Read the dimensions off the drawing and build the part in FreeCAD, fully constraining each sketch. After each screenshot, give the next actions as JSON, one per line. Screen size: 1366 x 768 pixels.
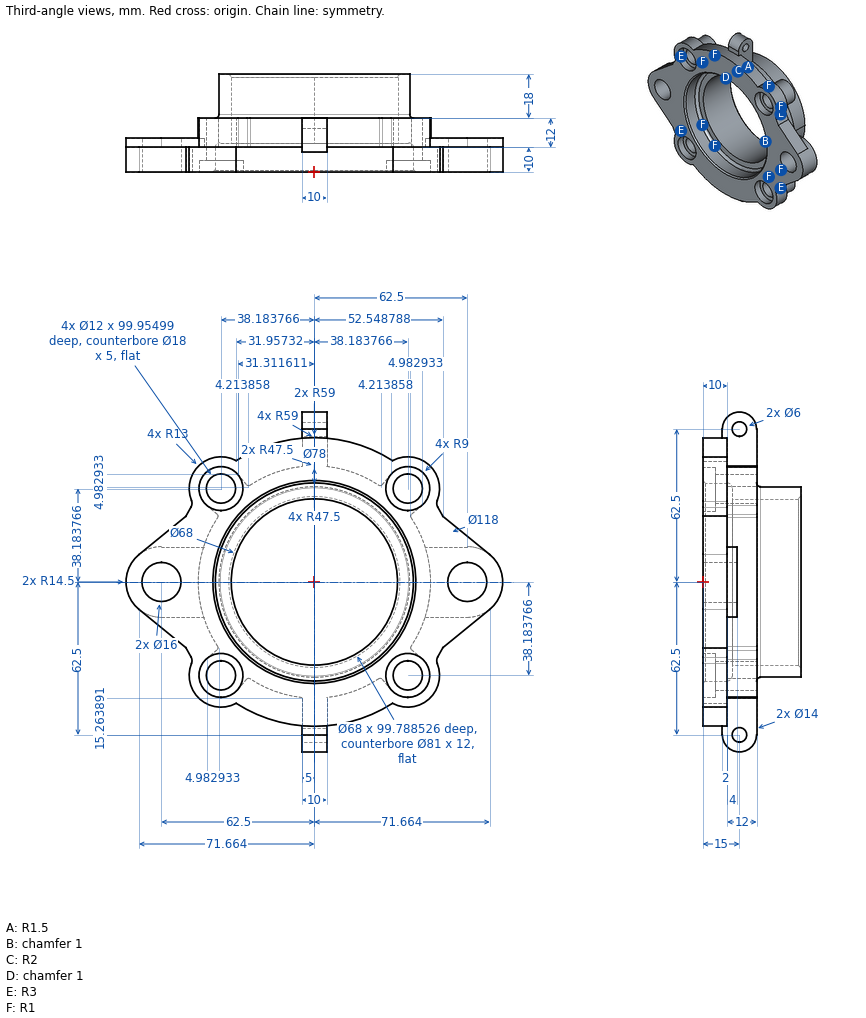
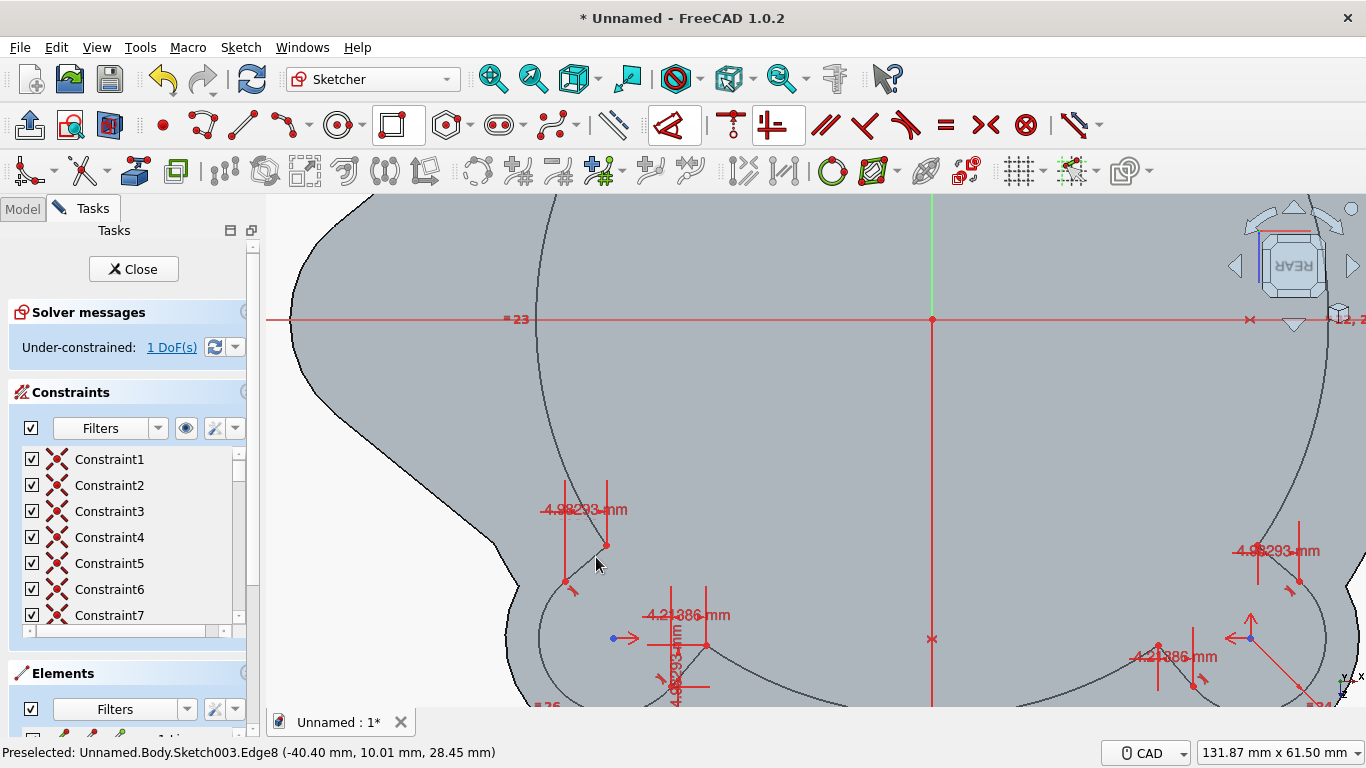
{"action": "scroll", "coordinate": [597, 557], "scroll_direction": "down", "scroll_amount": 4}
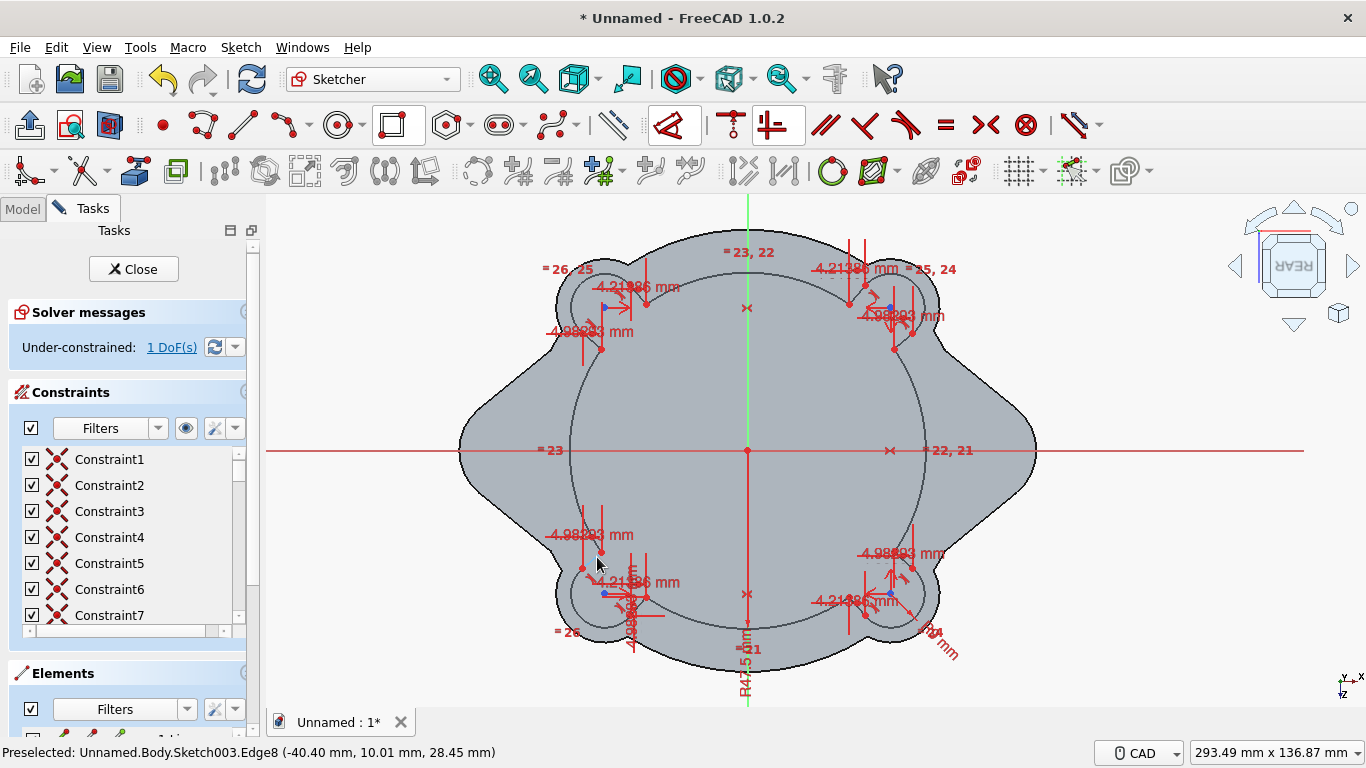
{"action": "left_click", "coordinate": [631, 616]}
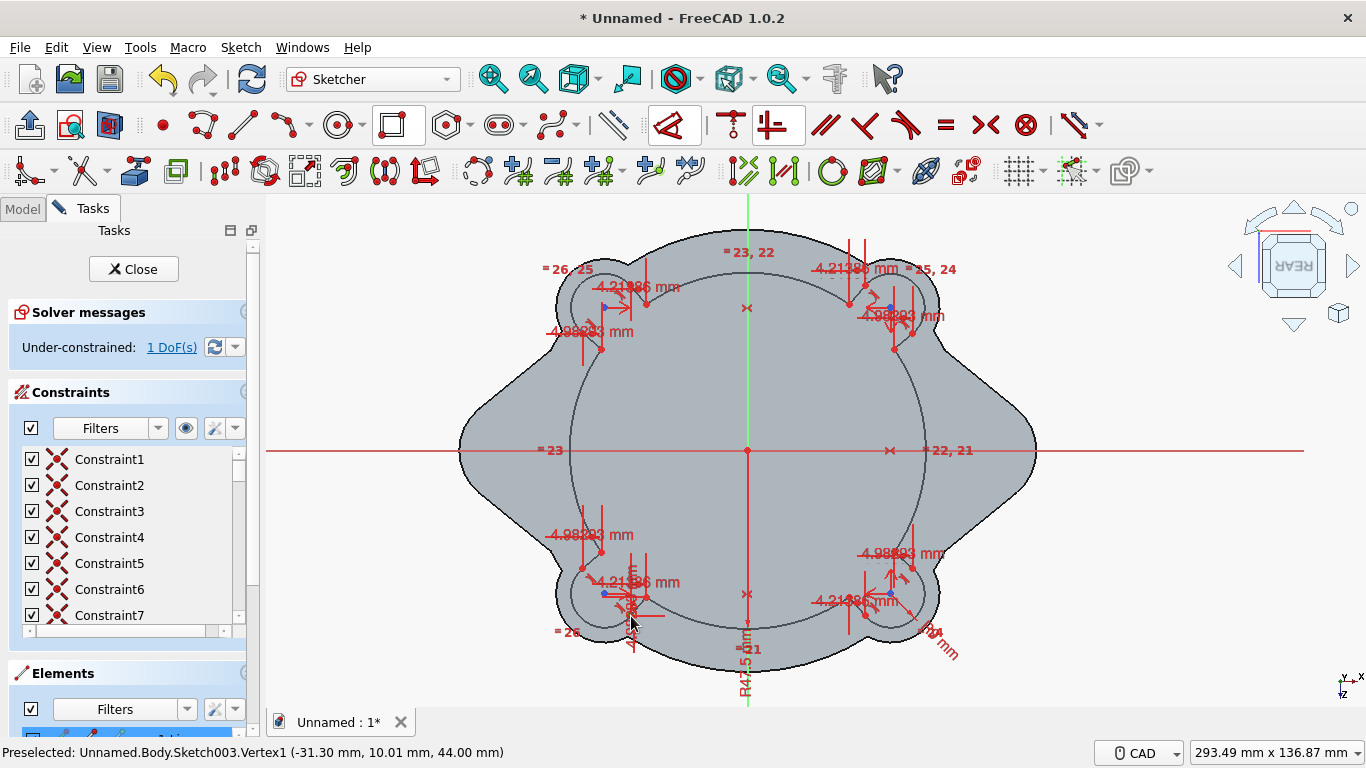
{"action": "key", "text": "l"}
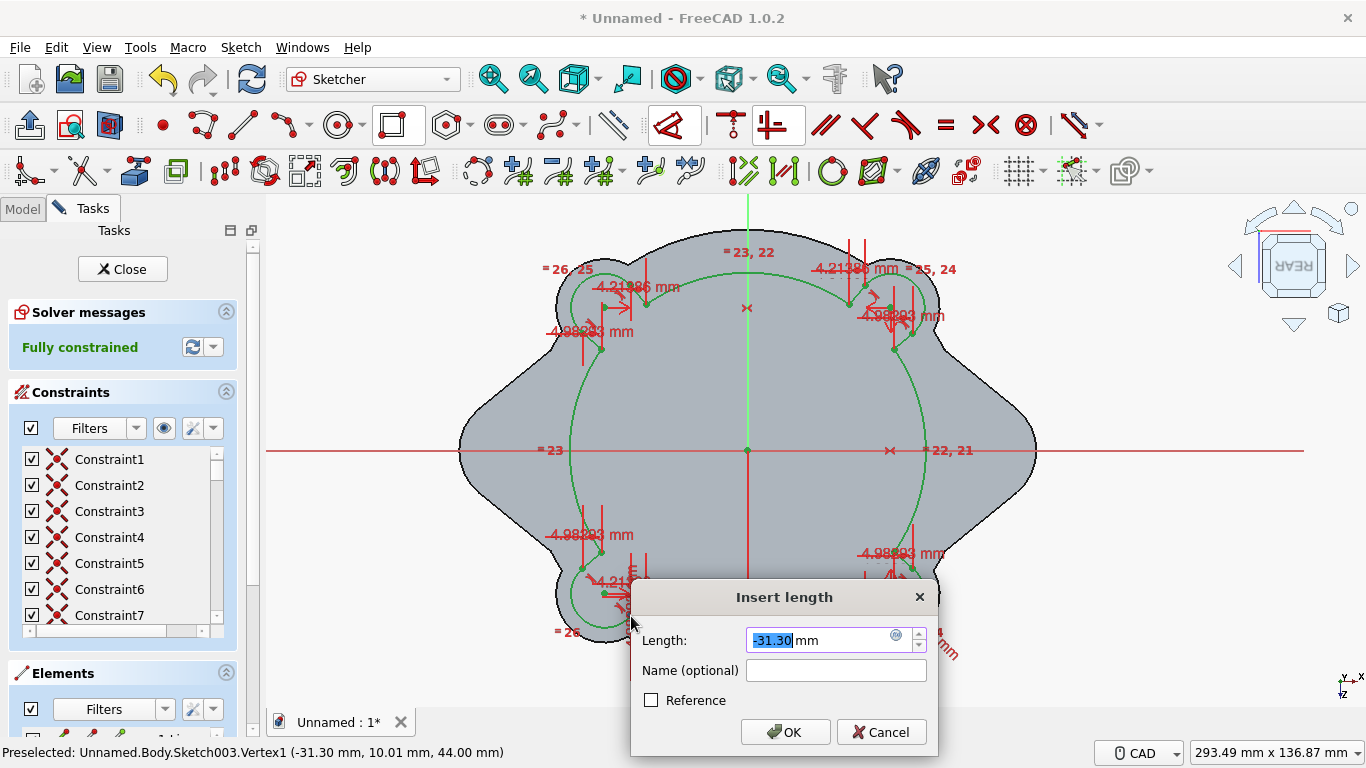
{"action": "type", "text": "-31.311611"}
{"action": "key", "text": "Return"}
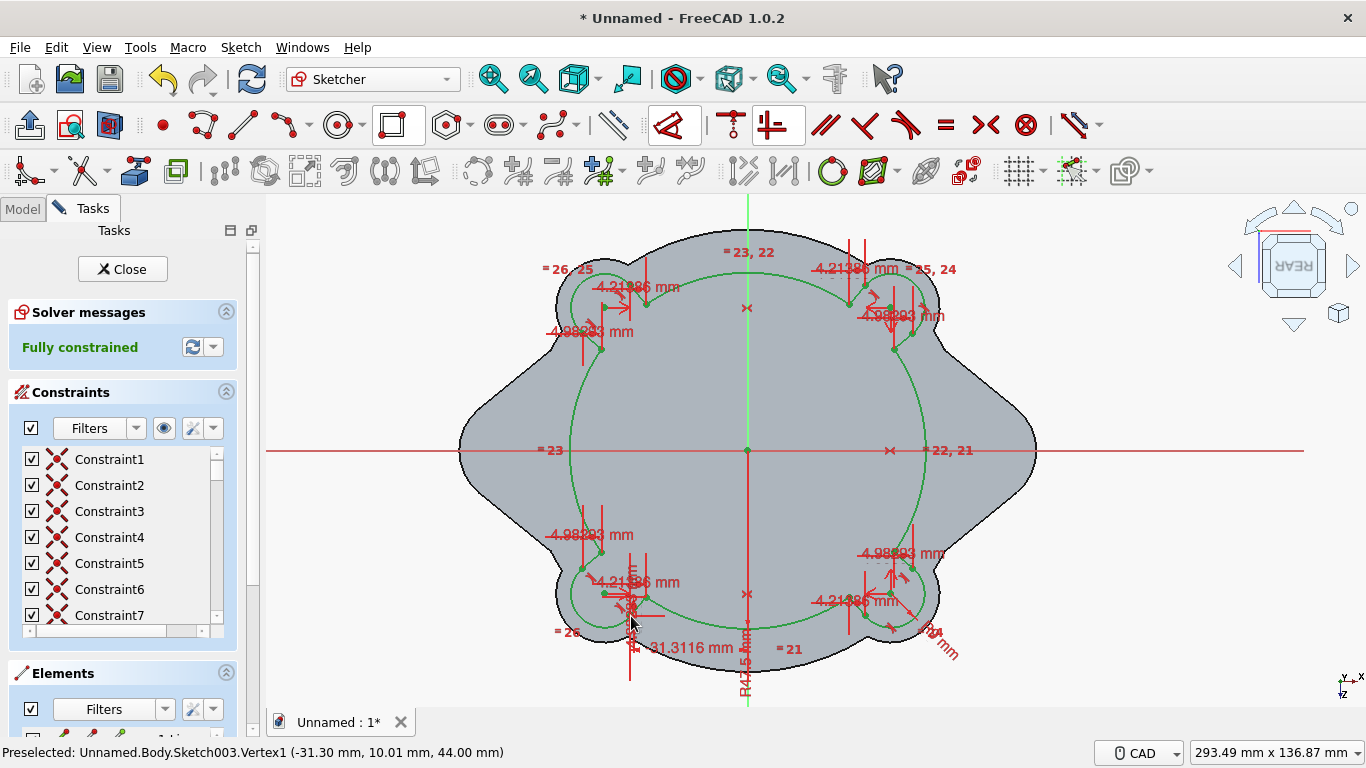
{"action": "left_click", "coordinate": [123, 269]}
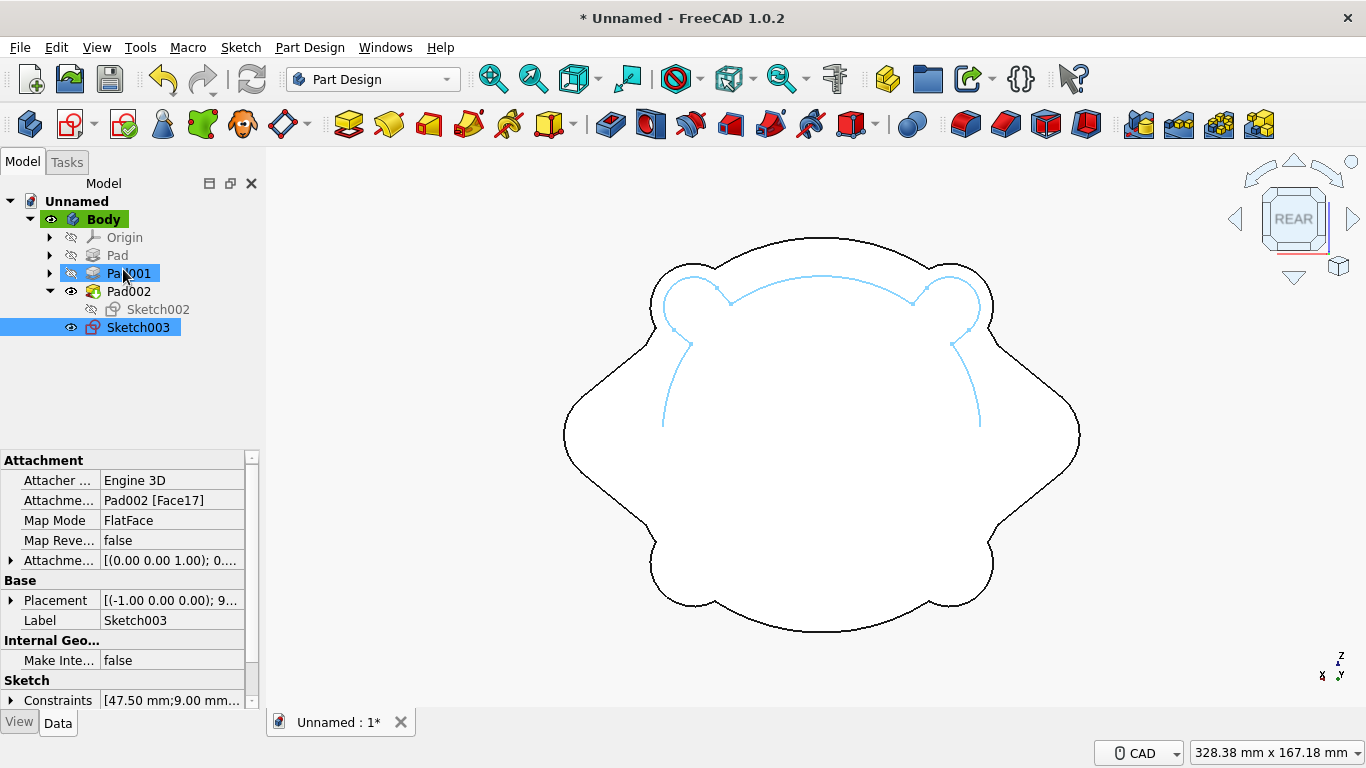
{"action": "left_click", "coordinate": [350, 124]}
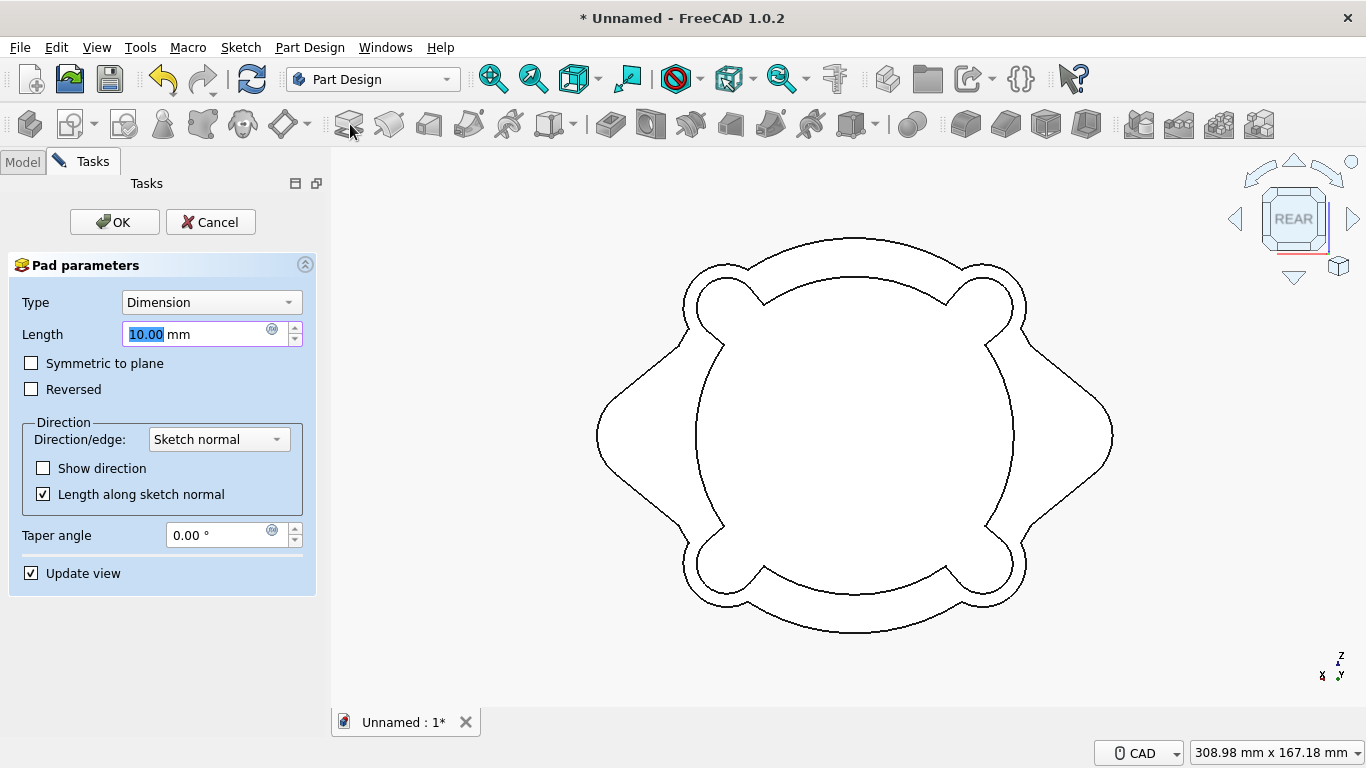
{"action": "type", "text": "12"}
{"action": "key", "text": "Tab"}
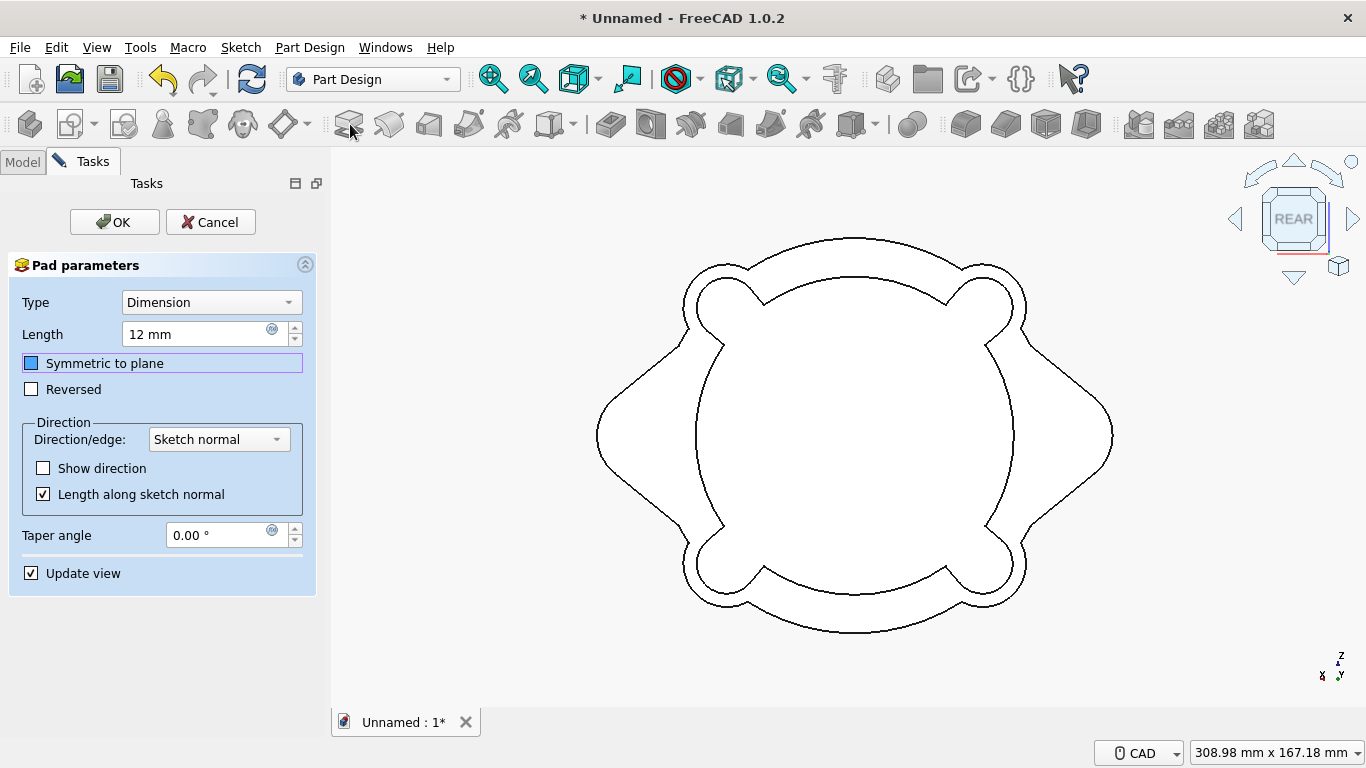
{"action": "left_click", "coordinate": [115, 222]}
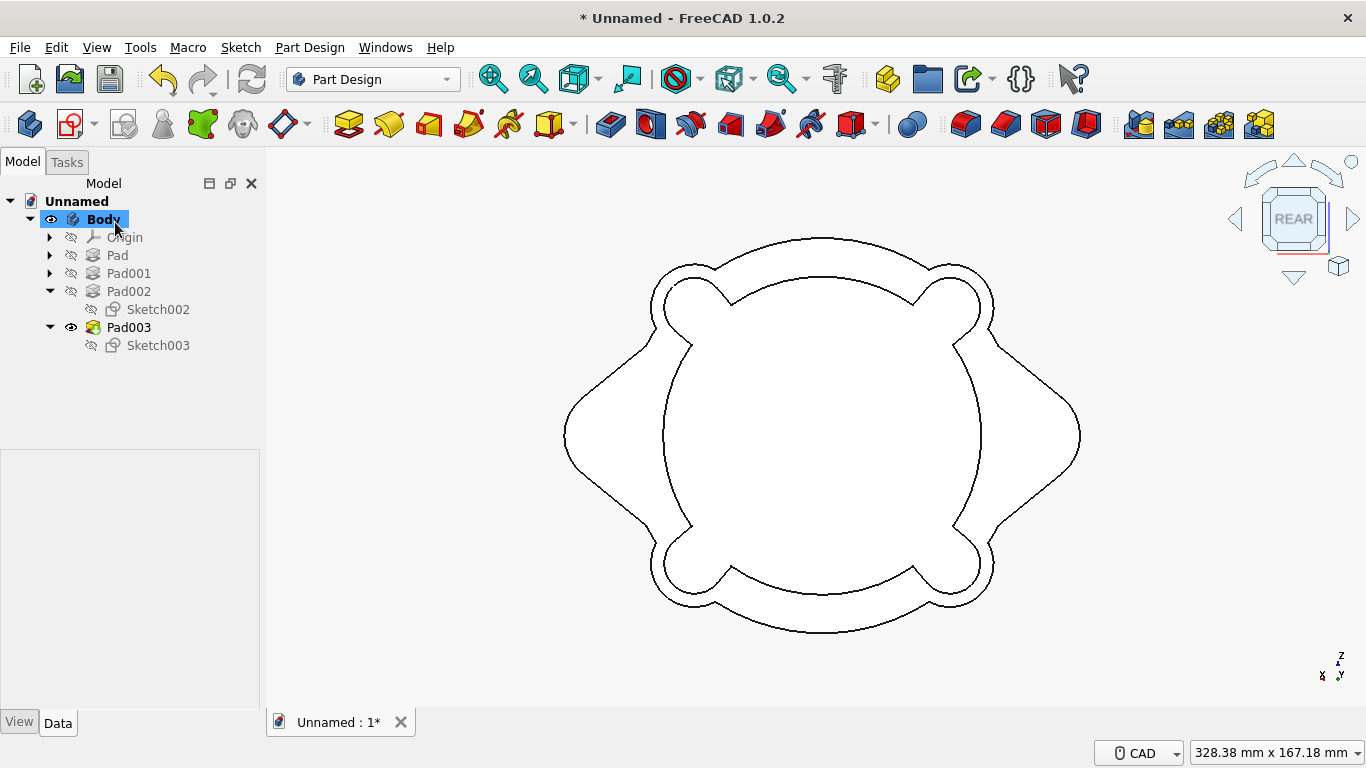
{"action": "left_click", "coordinate": [1043, 435]}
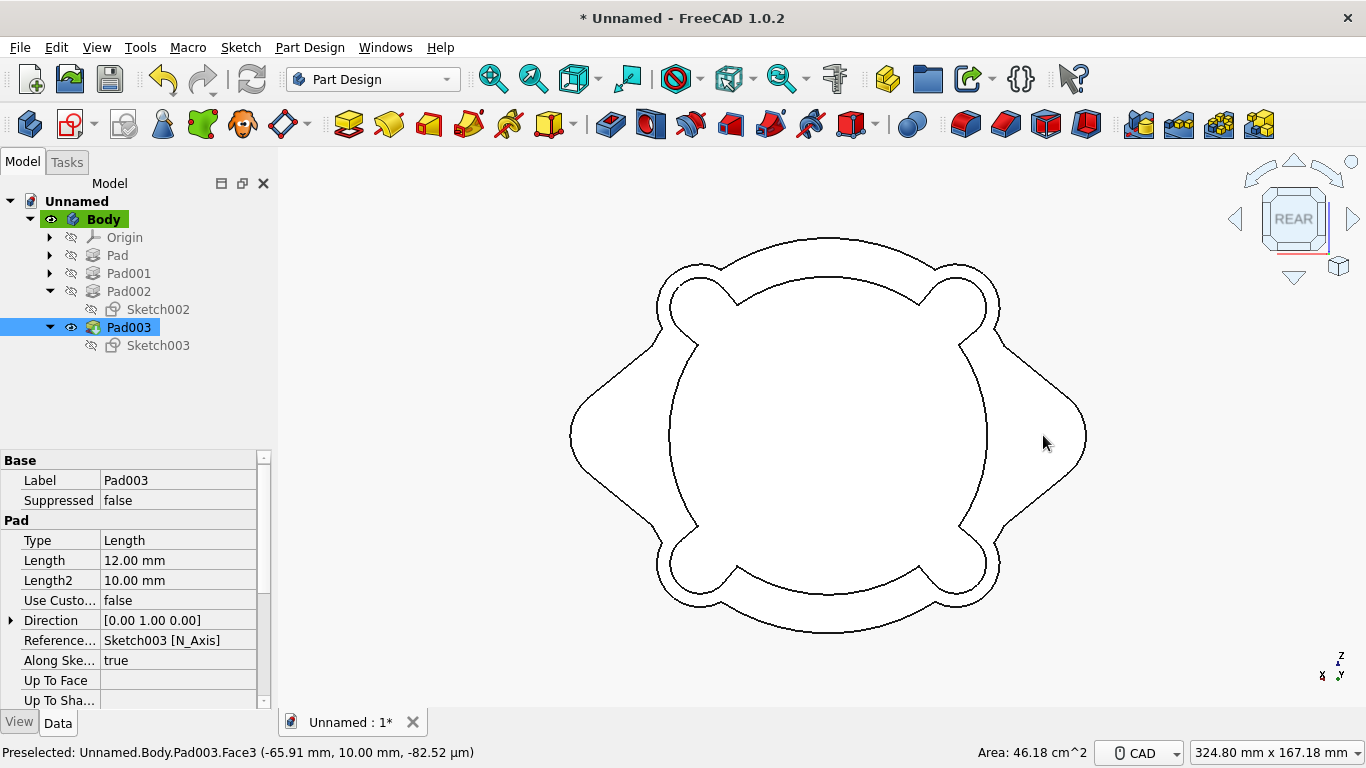
{"action": "left_click", "coordinate": [70, 124]}